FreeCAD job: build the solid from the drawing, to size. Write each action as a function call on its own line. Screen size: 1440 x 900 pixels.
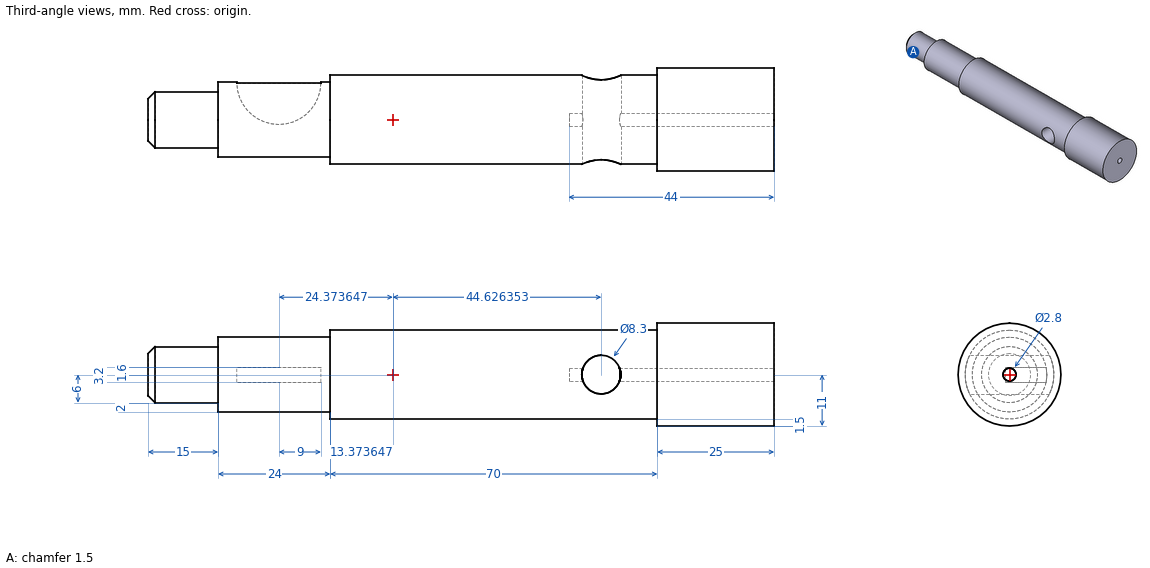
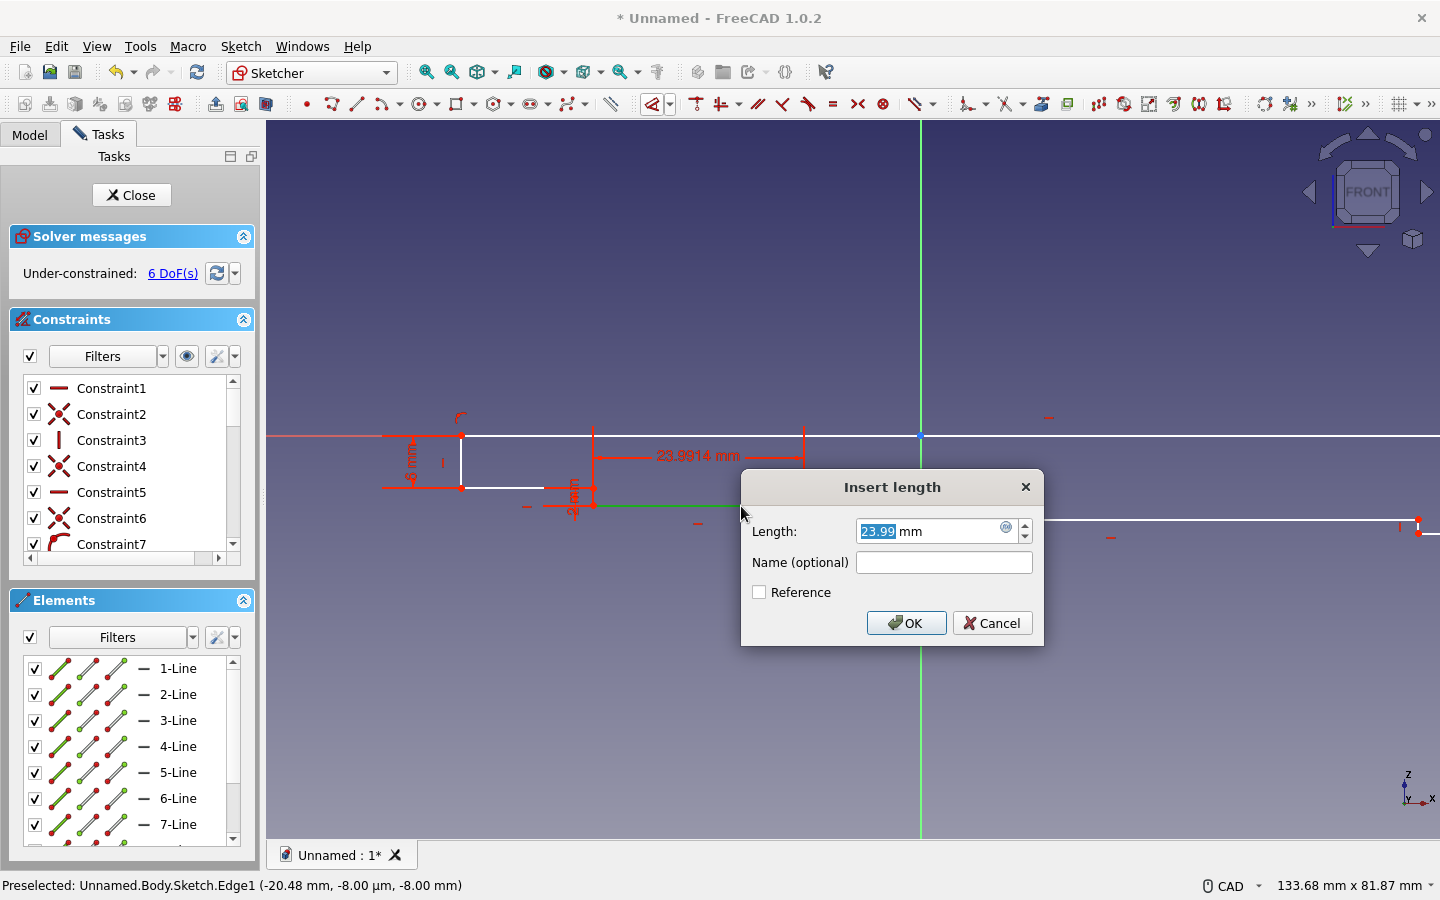
text(24)
key(Return)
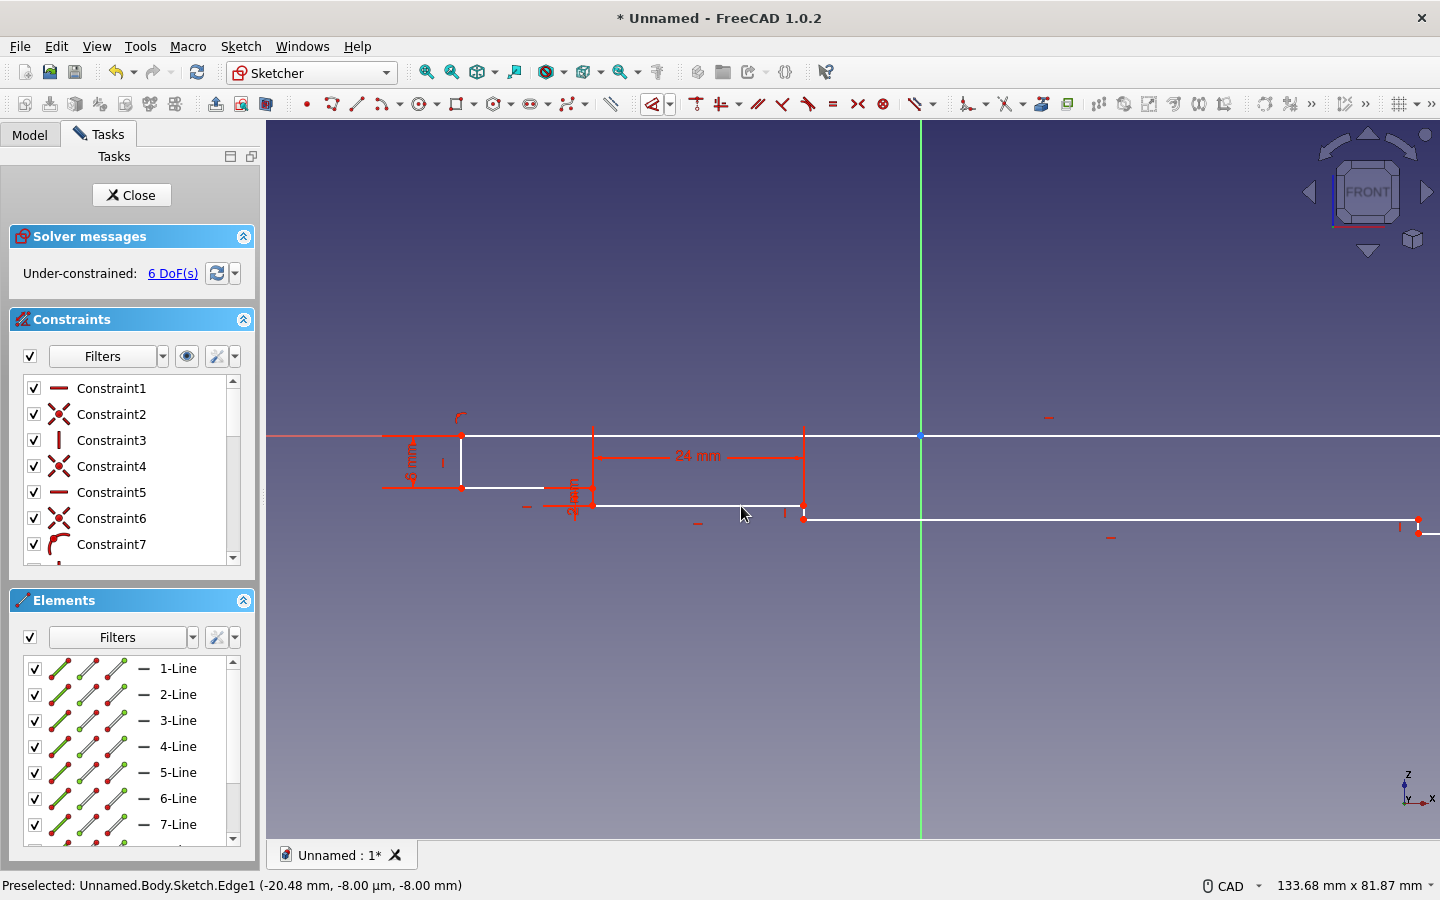
click(553, 488)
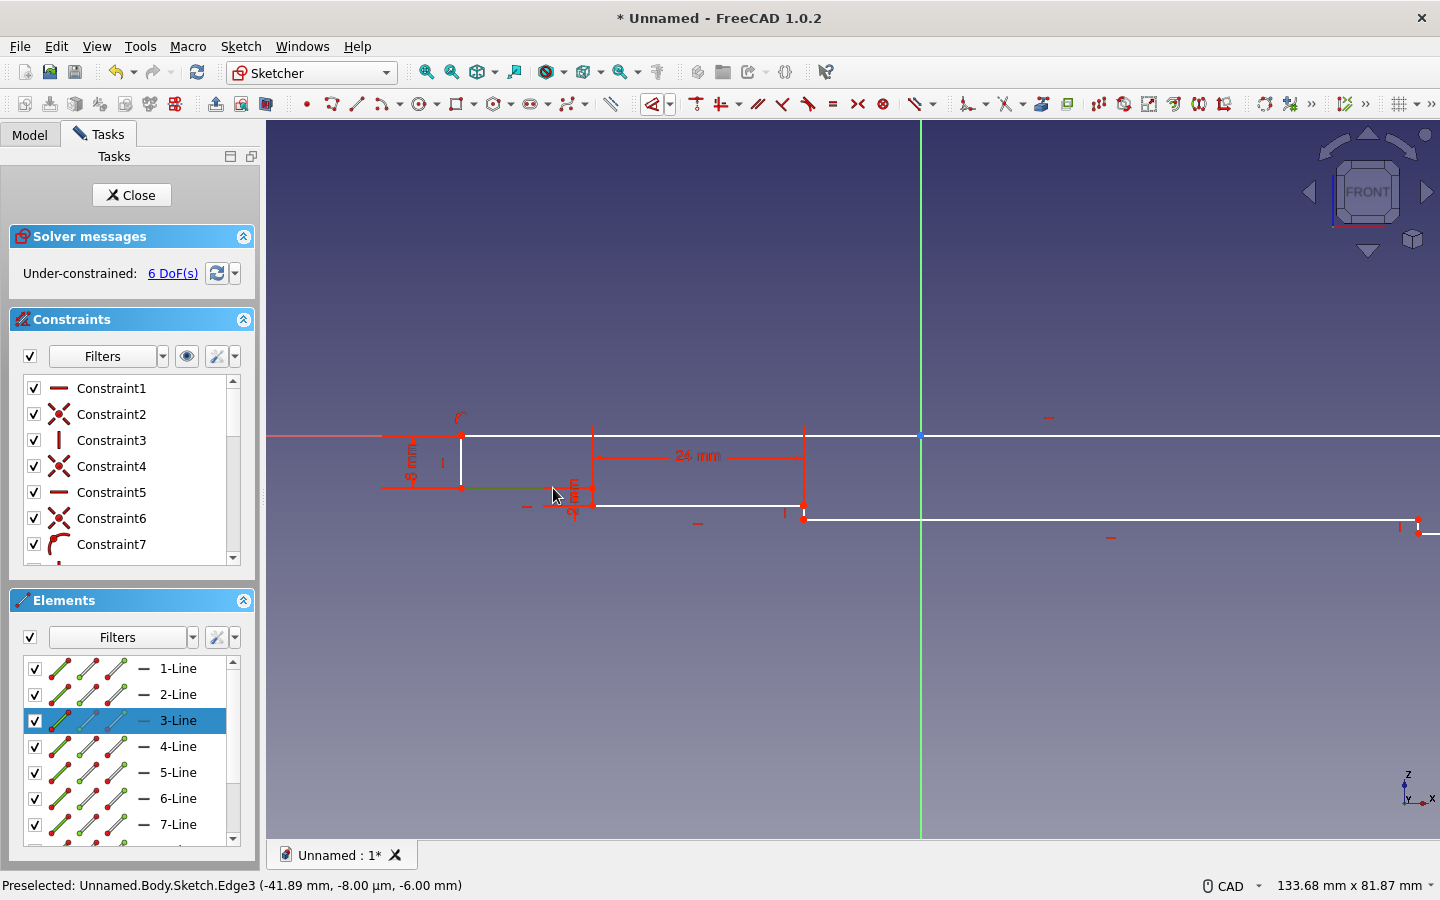
key(l)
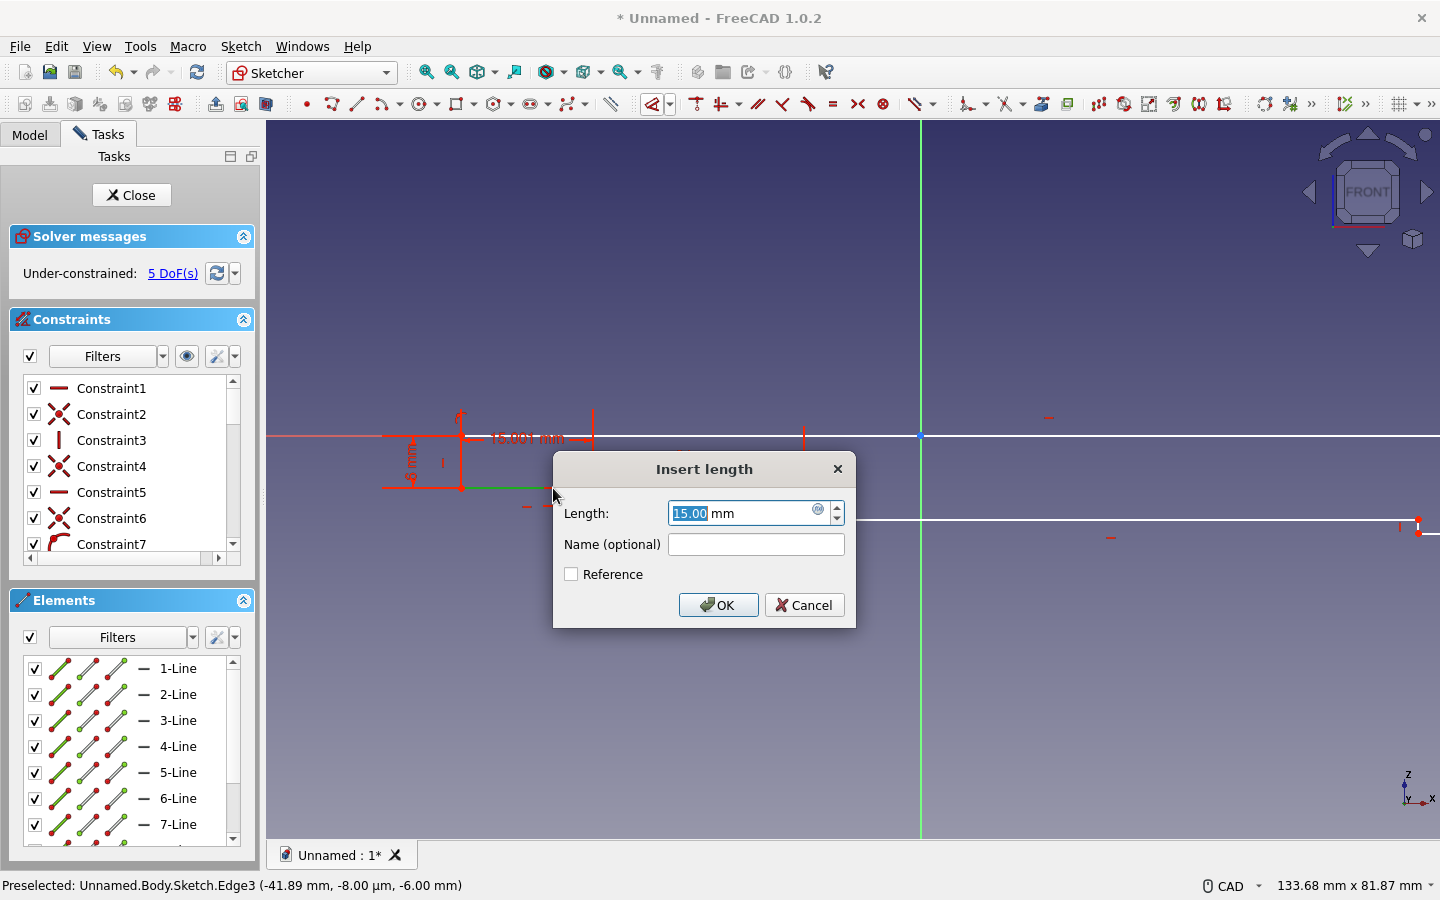
text(15)
key(Return)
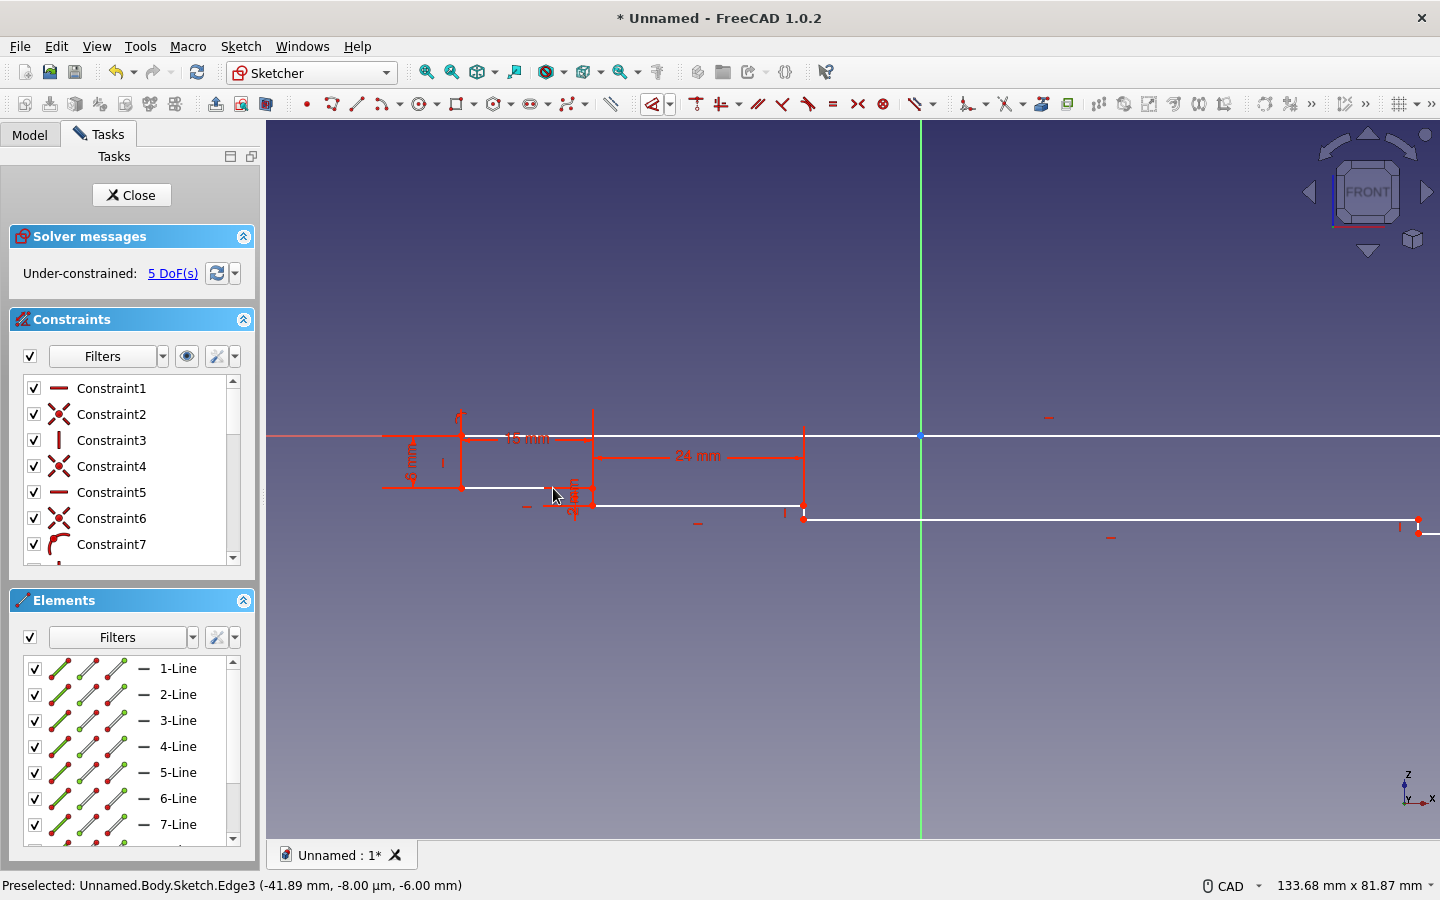
scroll(462, 474, down, 3)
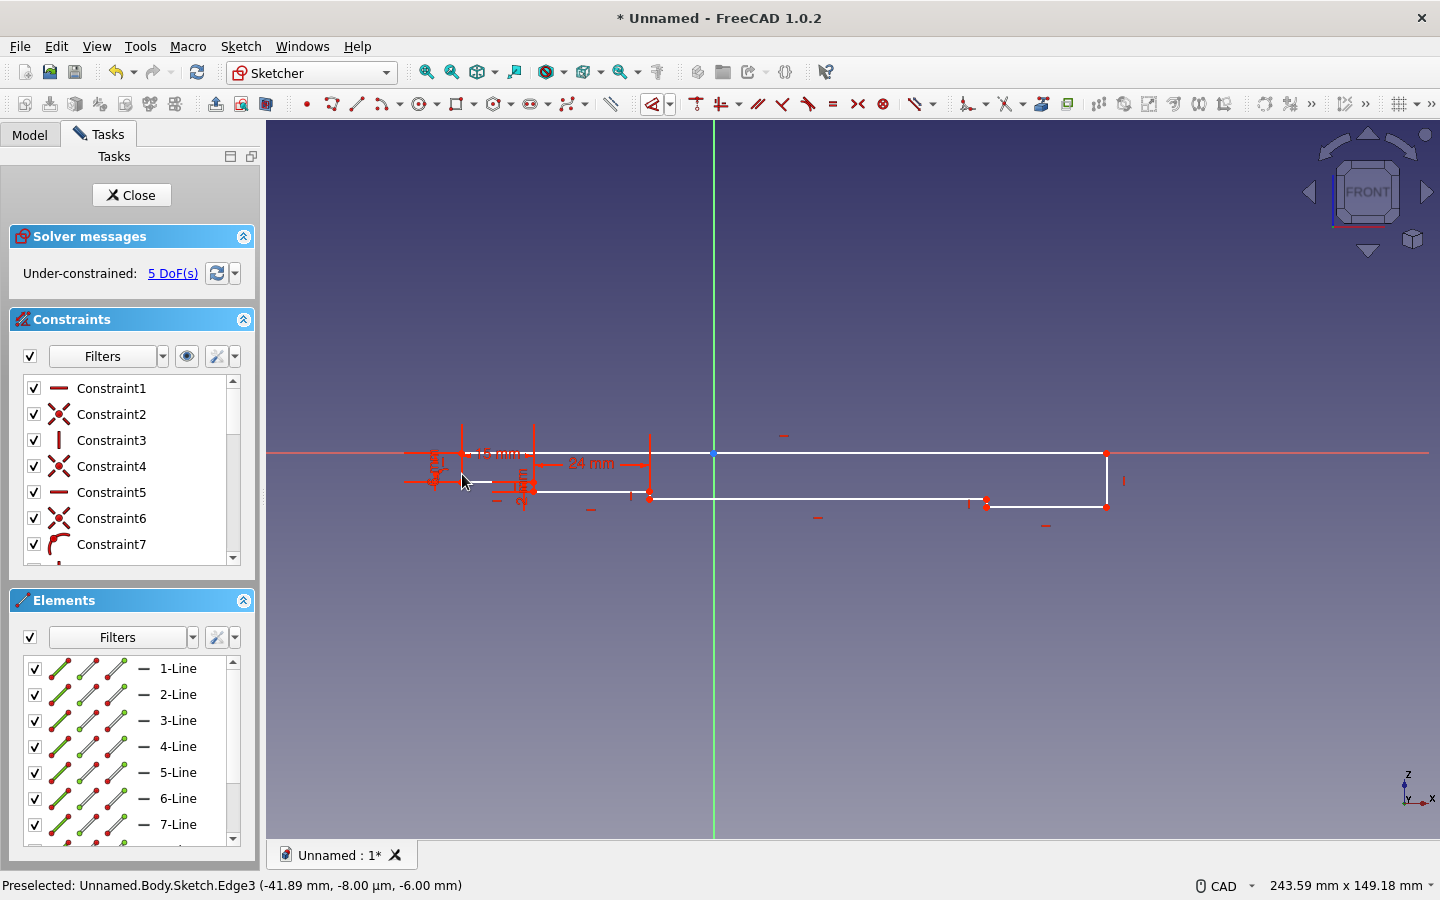
click(1107, 469)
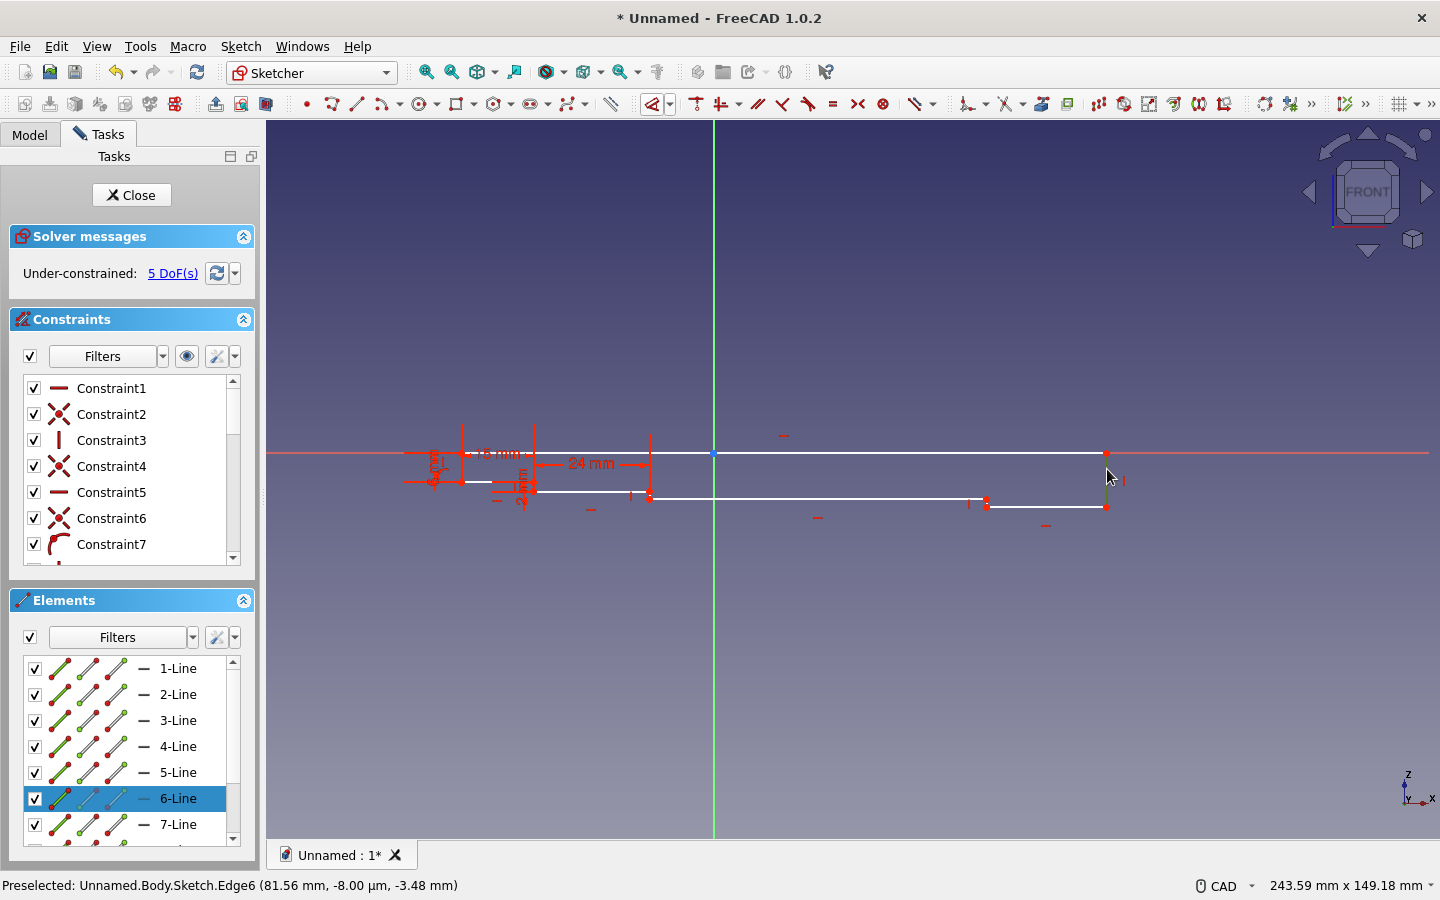
click(670, 104)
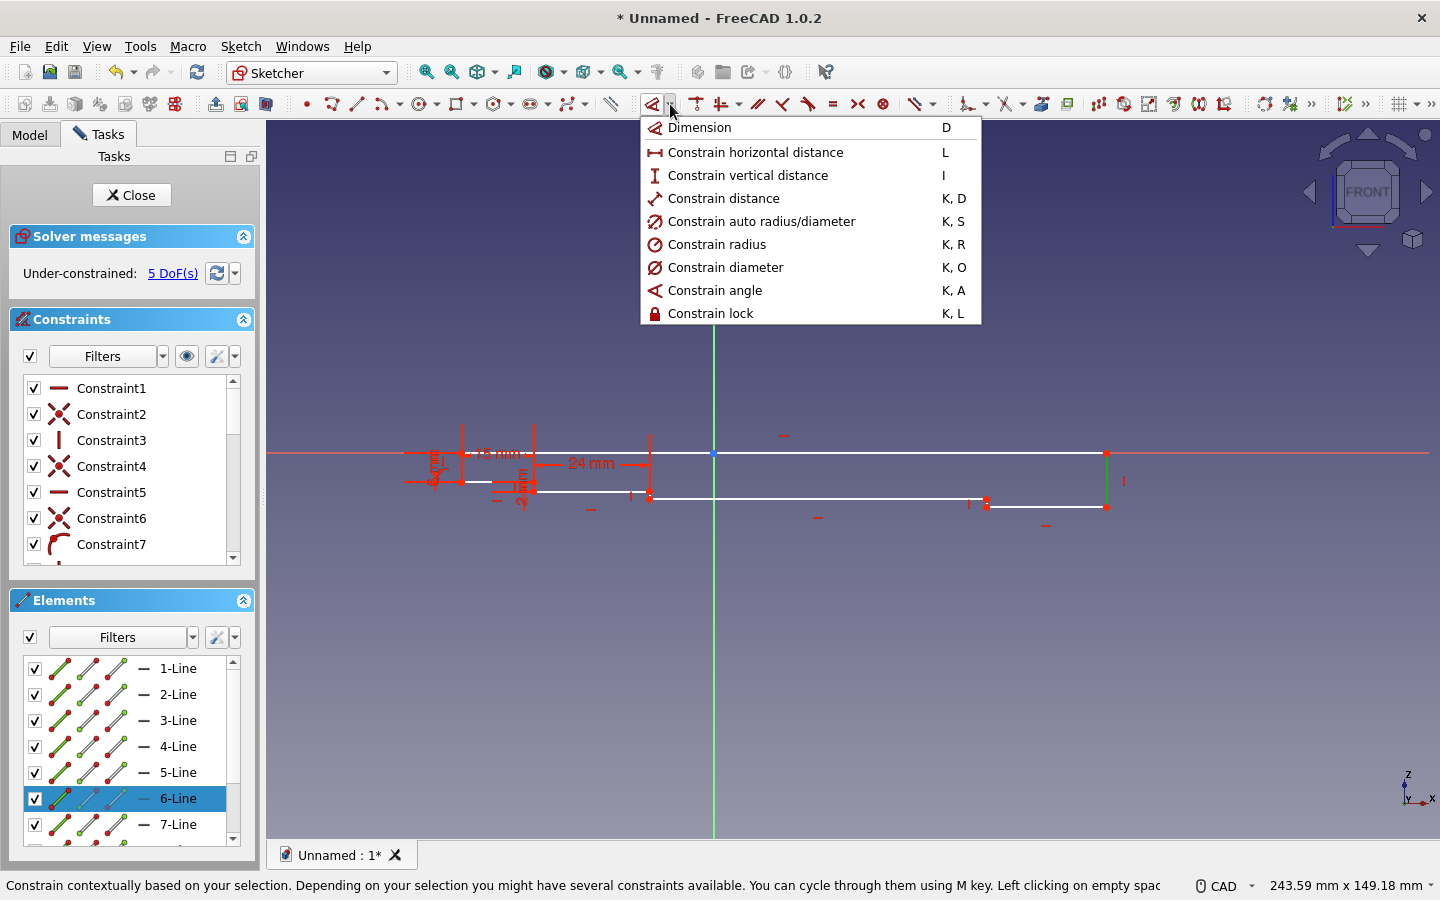
click(811, 176)